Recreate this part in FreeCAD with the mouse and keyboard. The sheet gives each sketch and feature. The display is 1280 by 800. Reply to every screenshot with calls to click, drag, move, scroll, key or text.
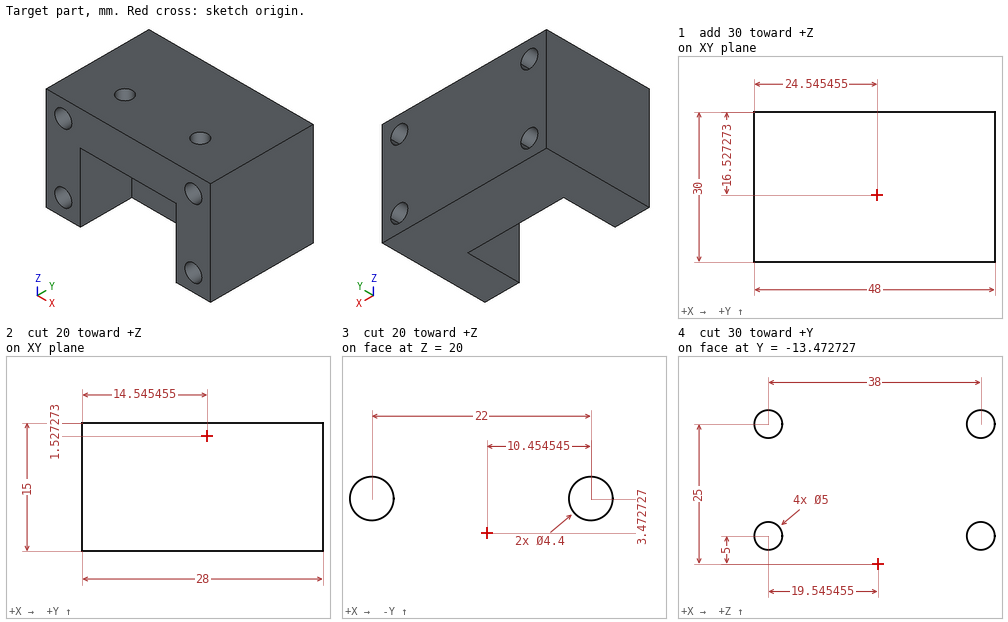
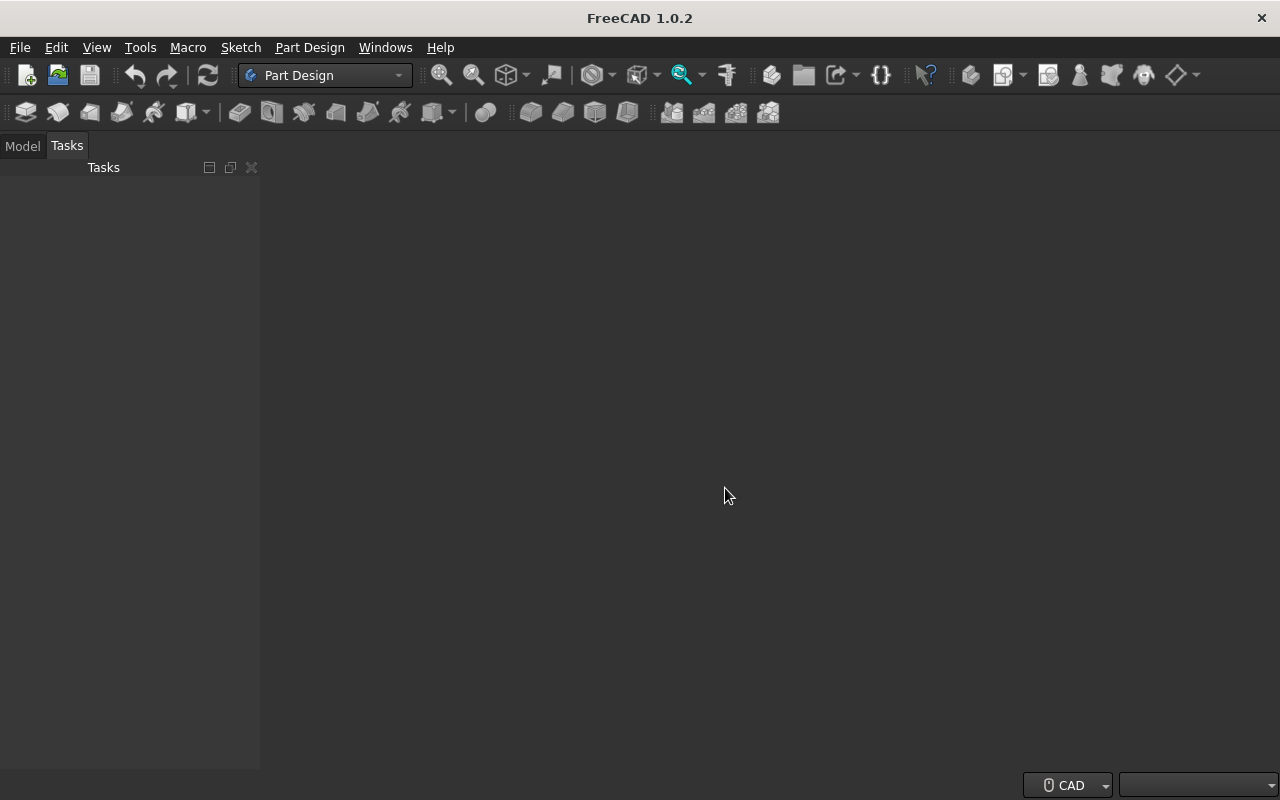
key(ctrl+n)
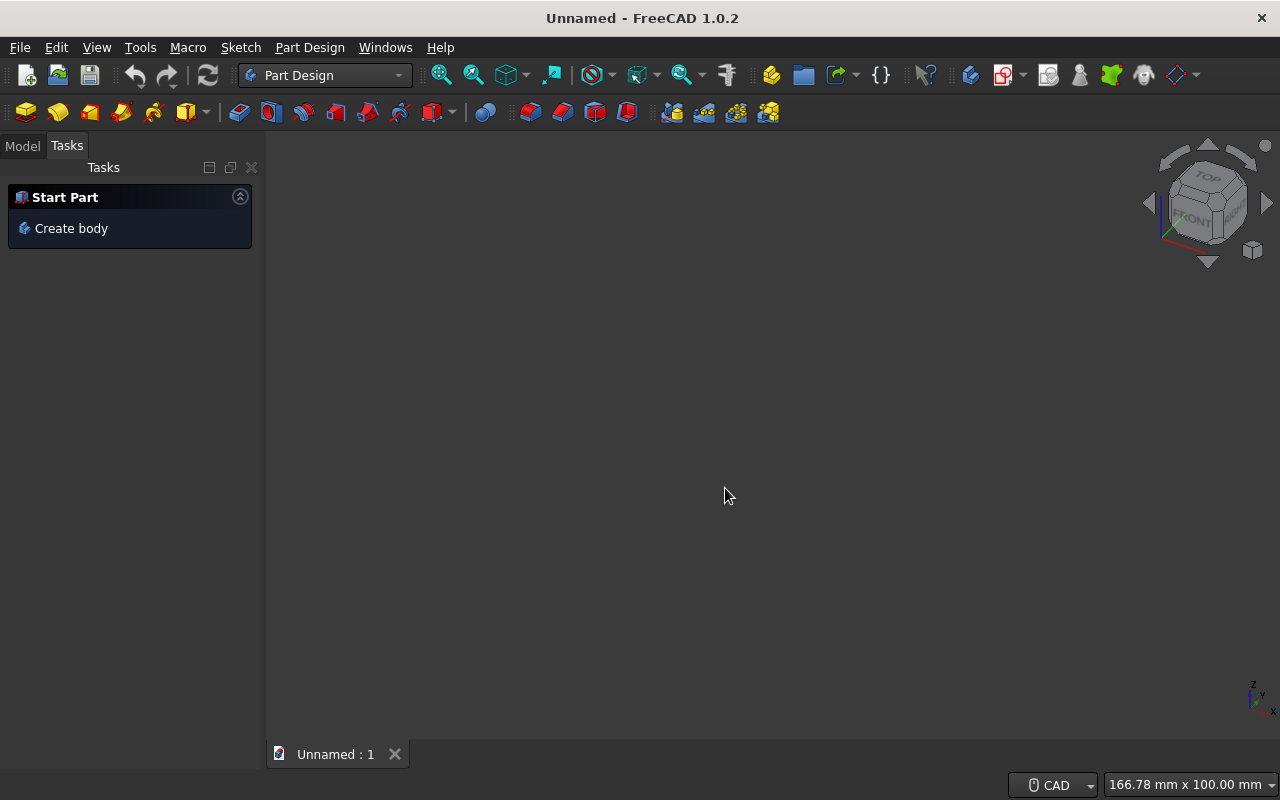
click(1004, 76)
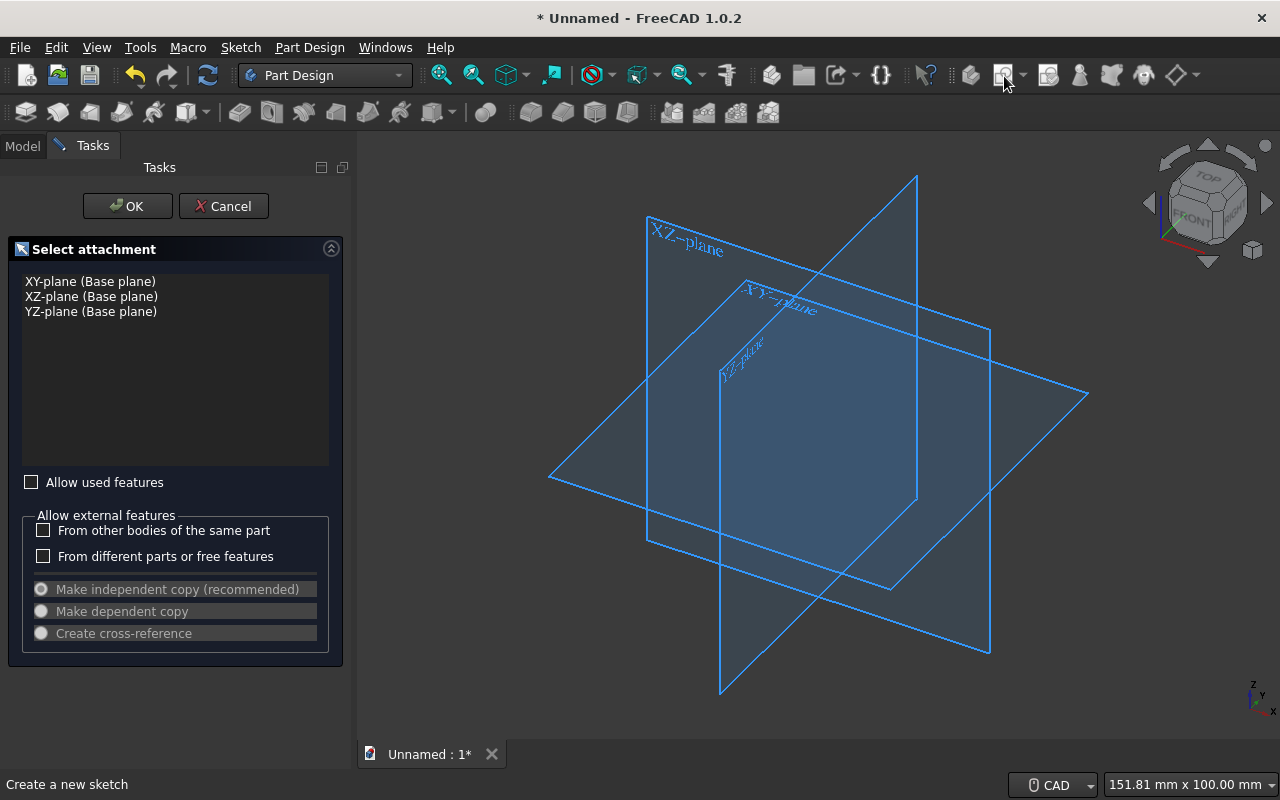
click(82, 282)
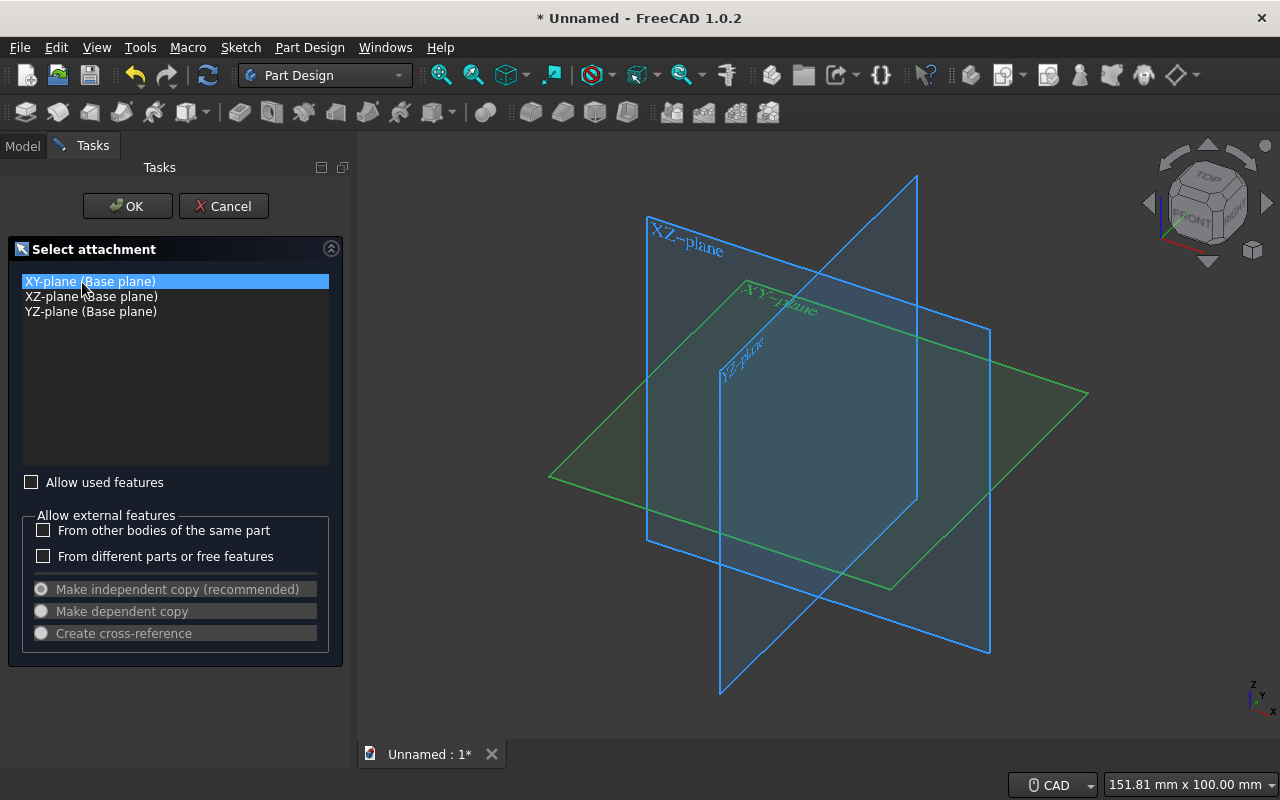
click(128, 206)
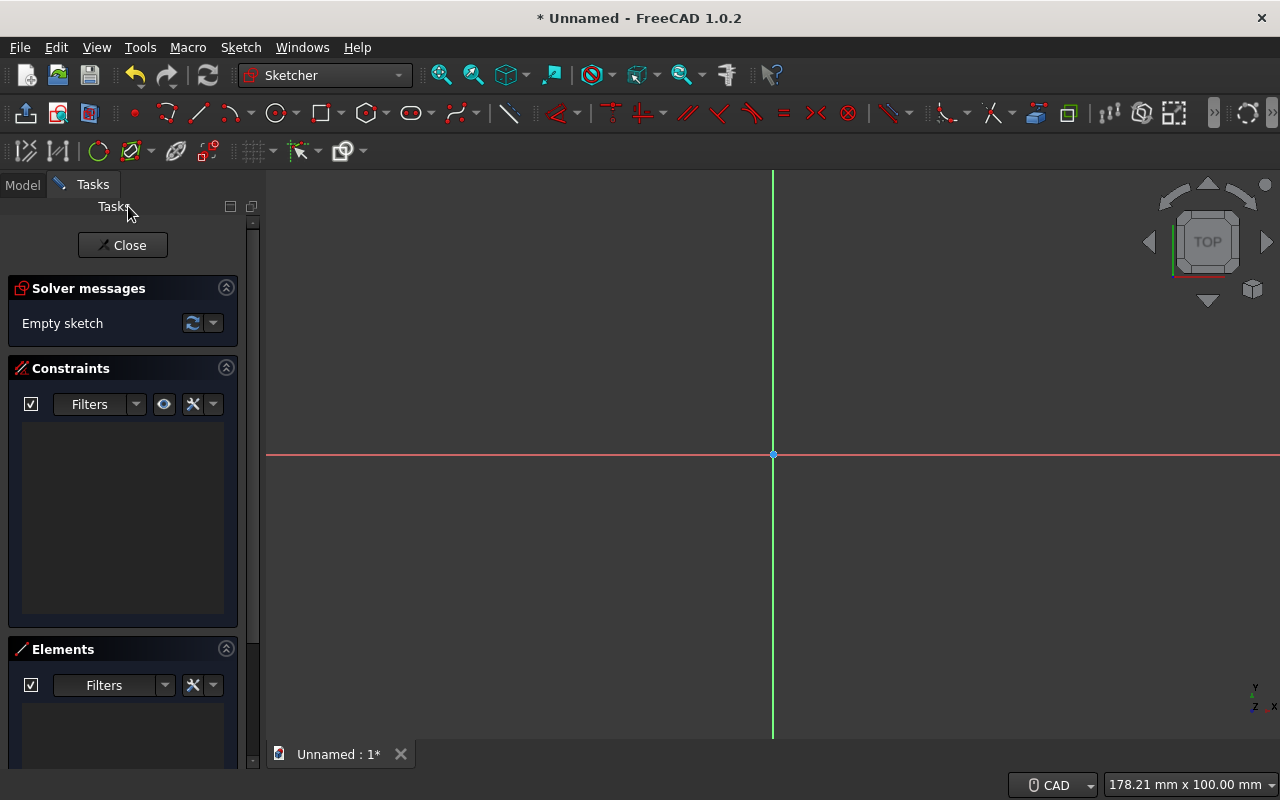
scroll(823, 439, up, 4)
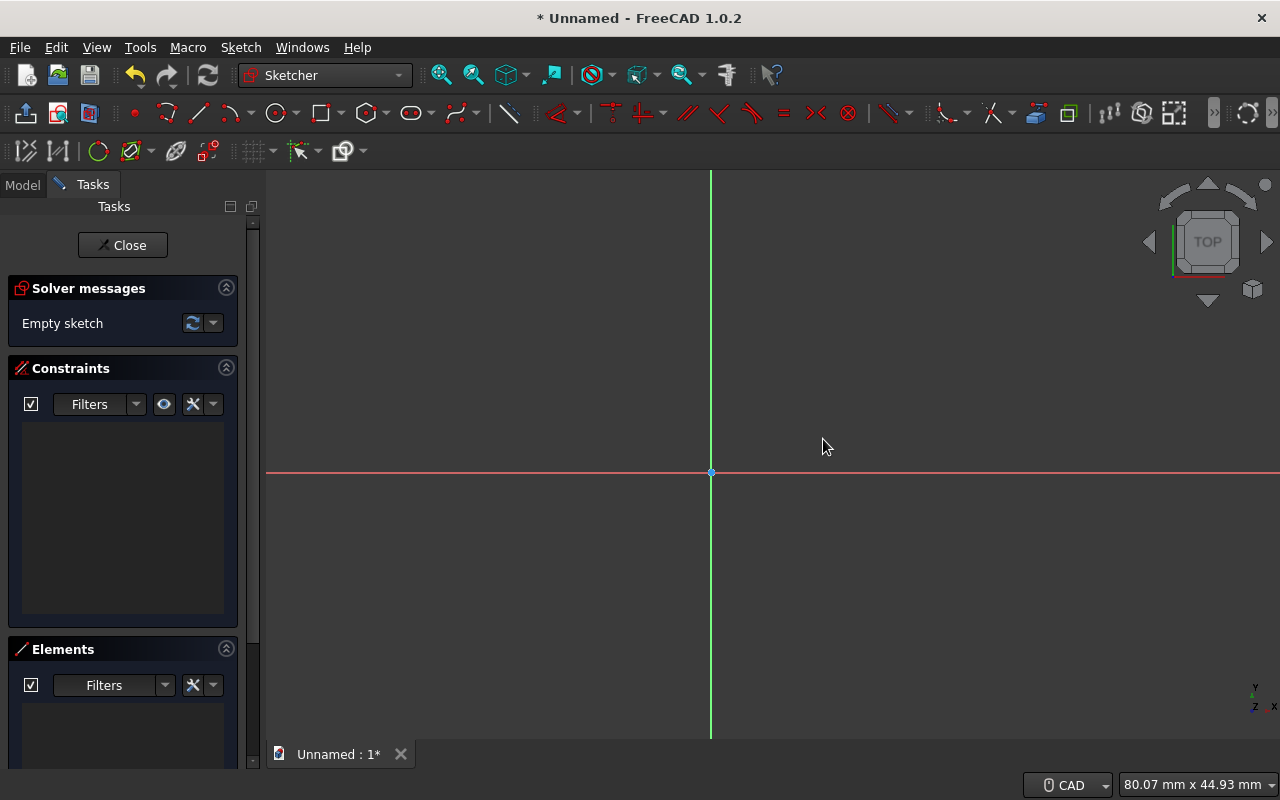
click(322, 114)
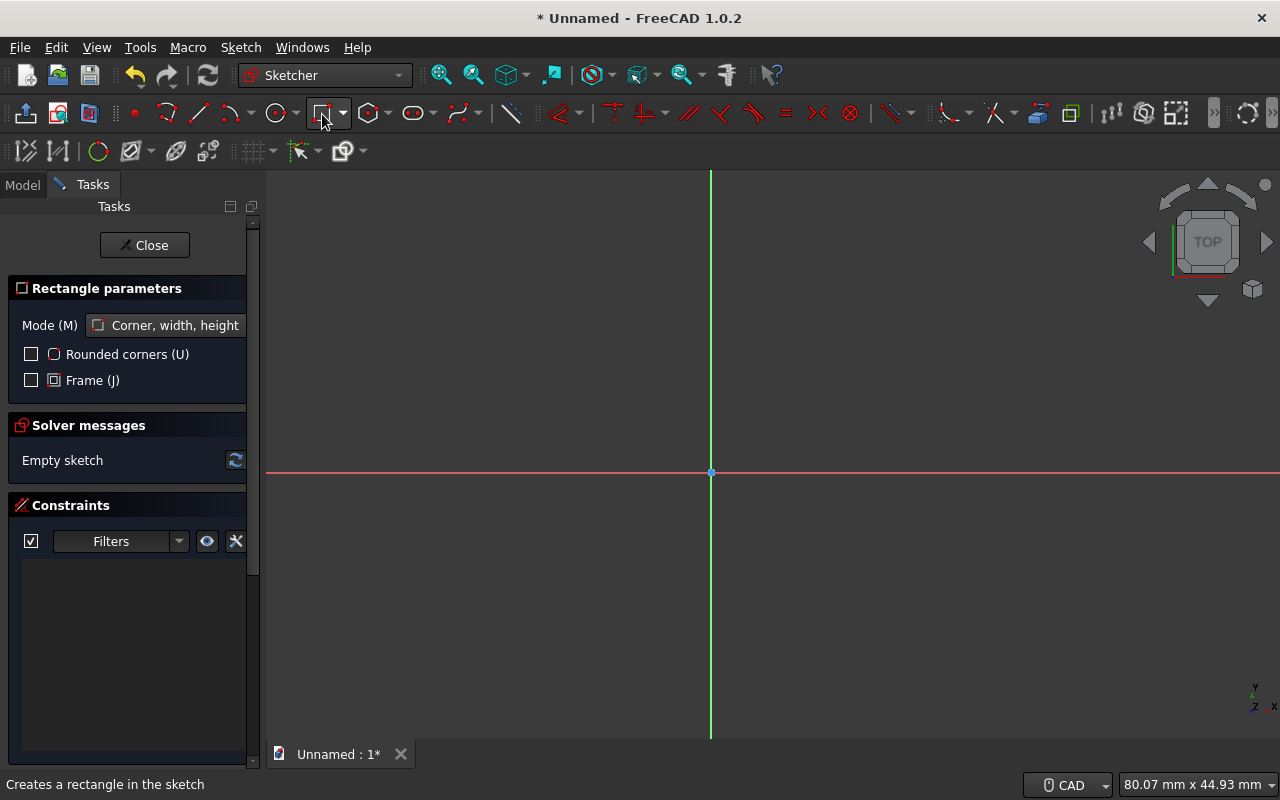
click(400, 264)
click(1008, 644)
key(Escape)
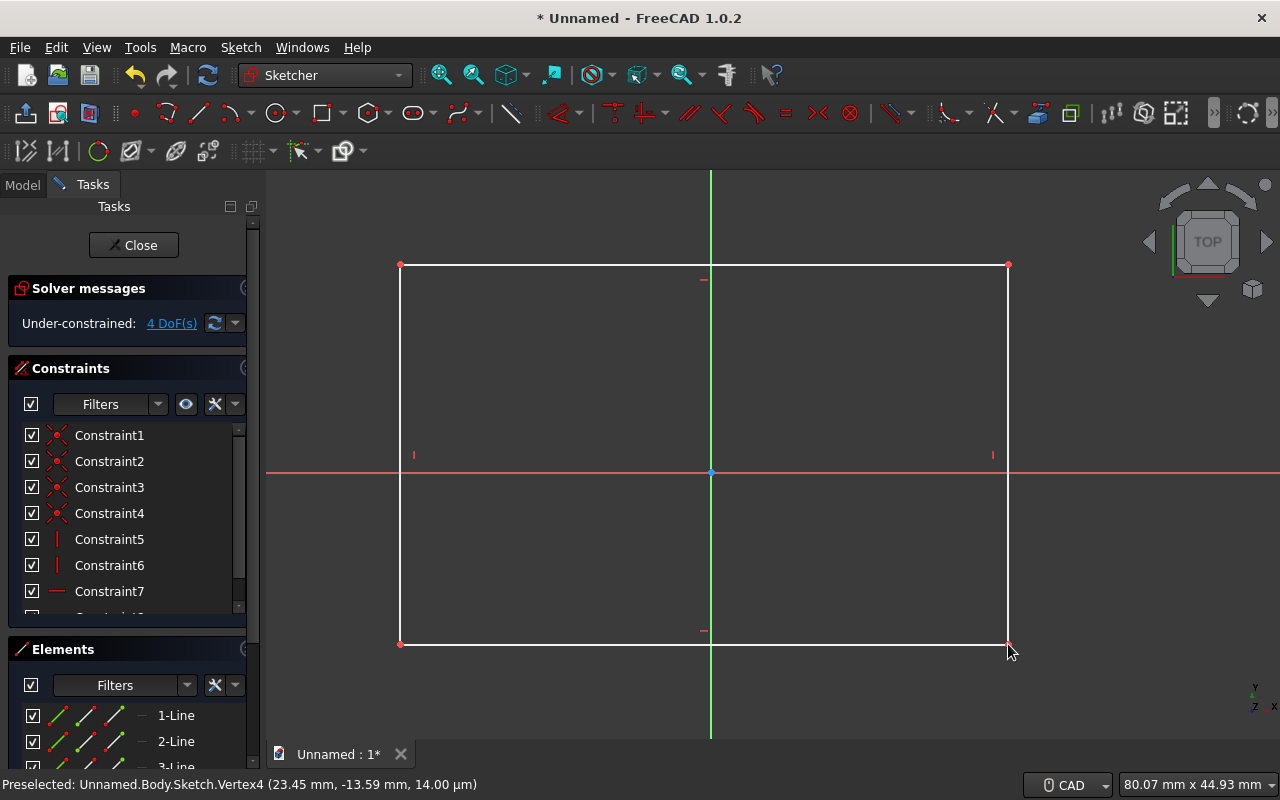
click(558, 114)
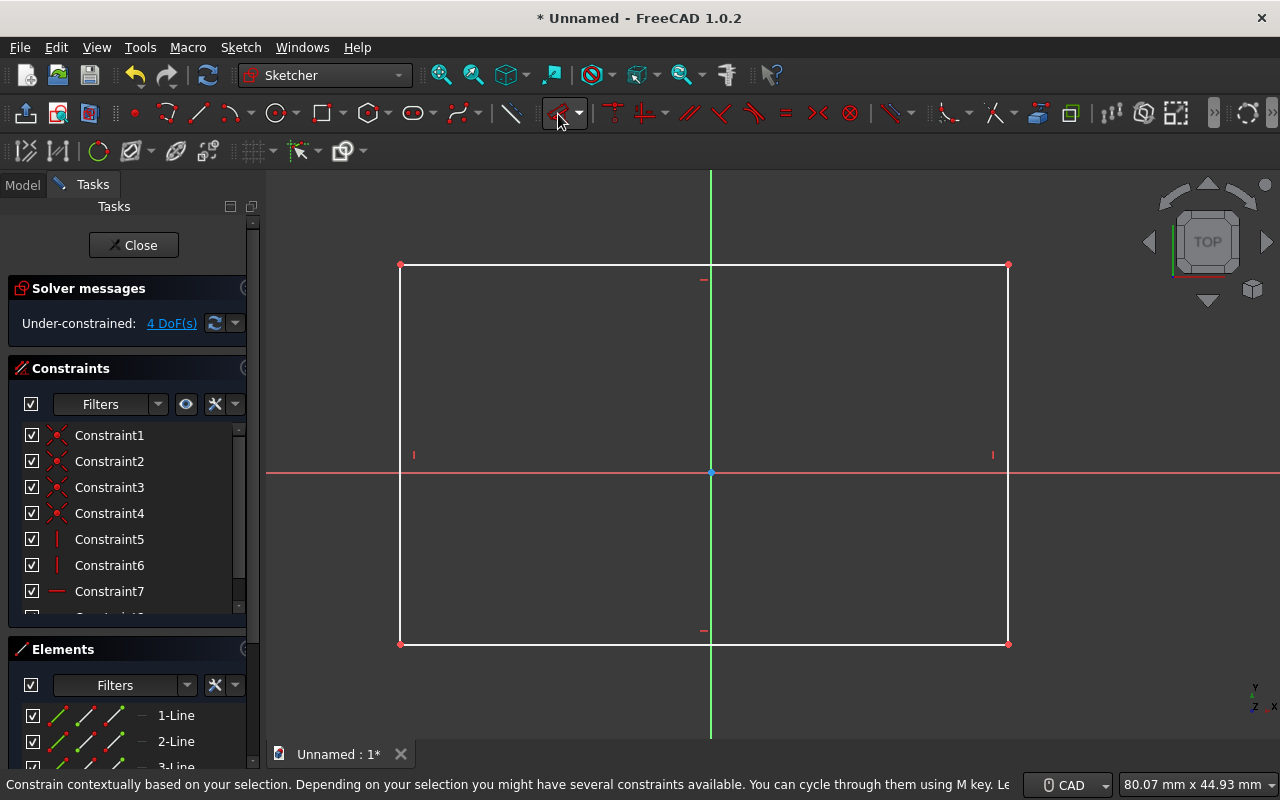
click(400, 379)
click(366, 455)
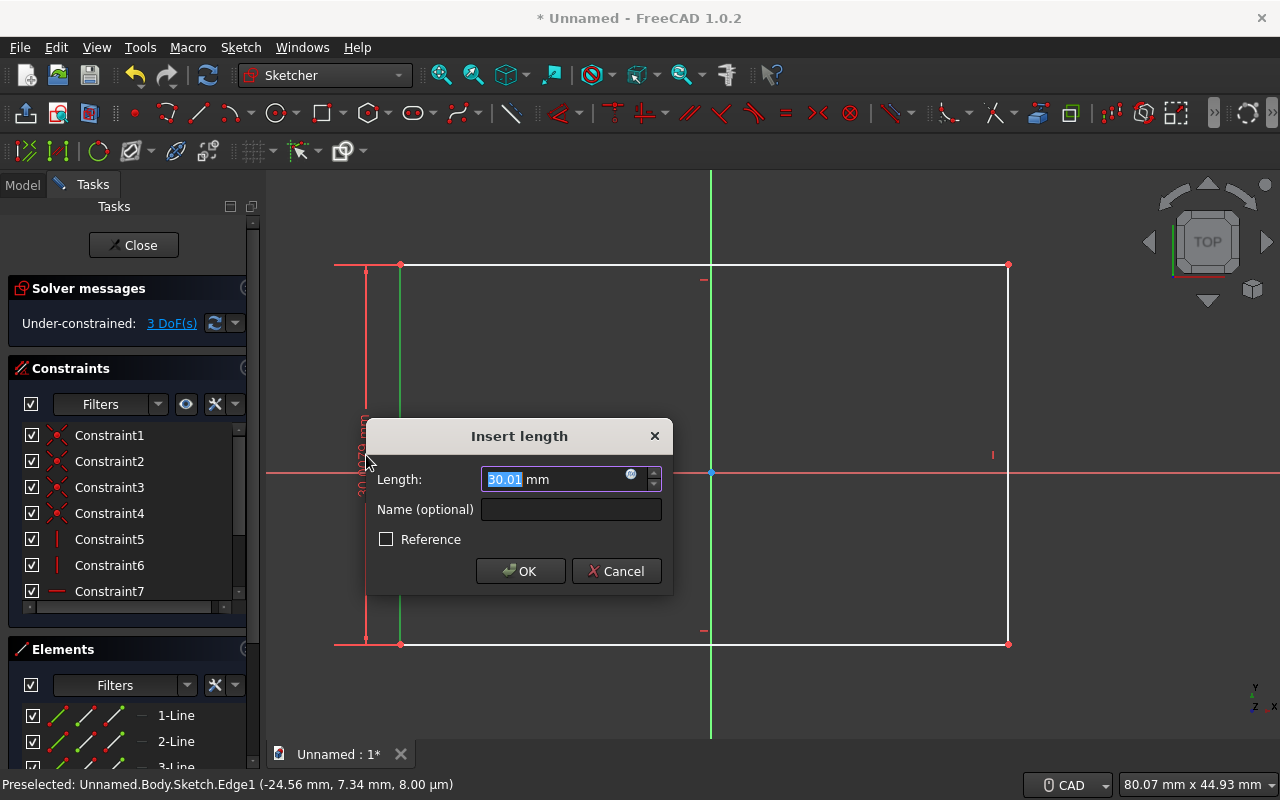
text(30)
key(Return)